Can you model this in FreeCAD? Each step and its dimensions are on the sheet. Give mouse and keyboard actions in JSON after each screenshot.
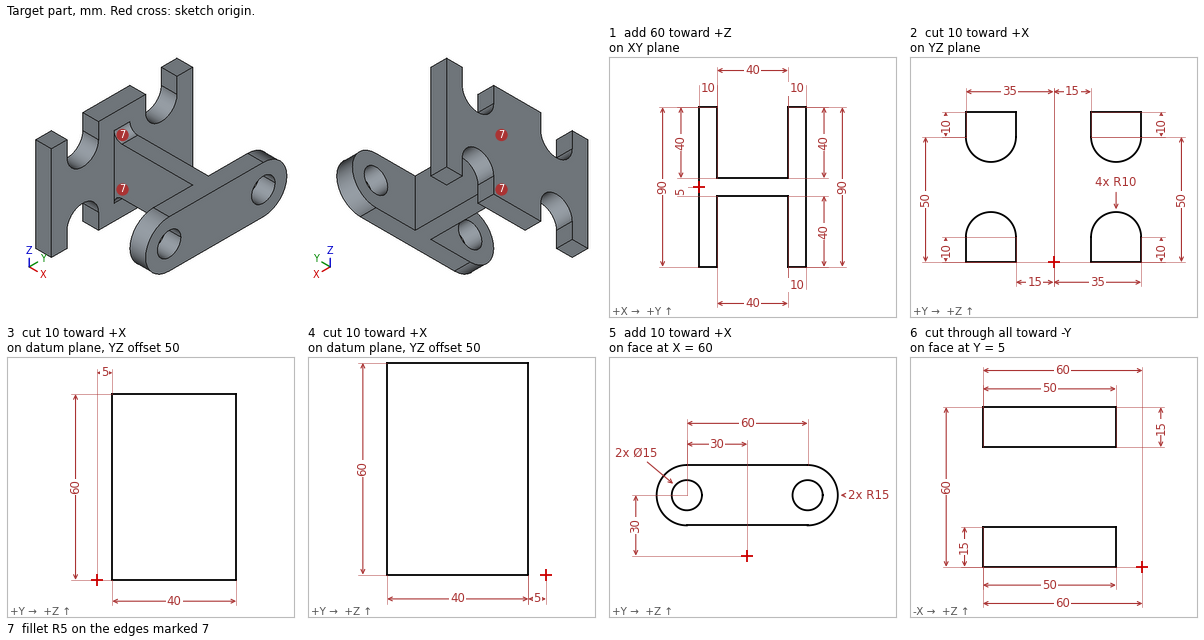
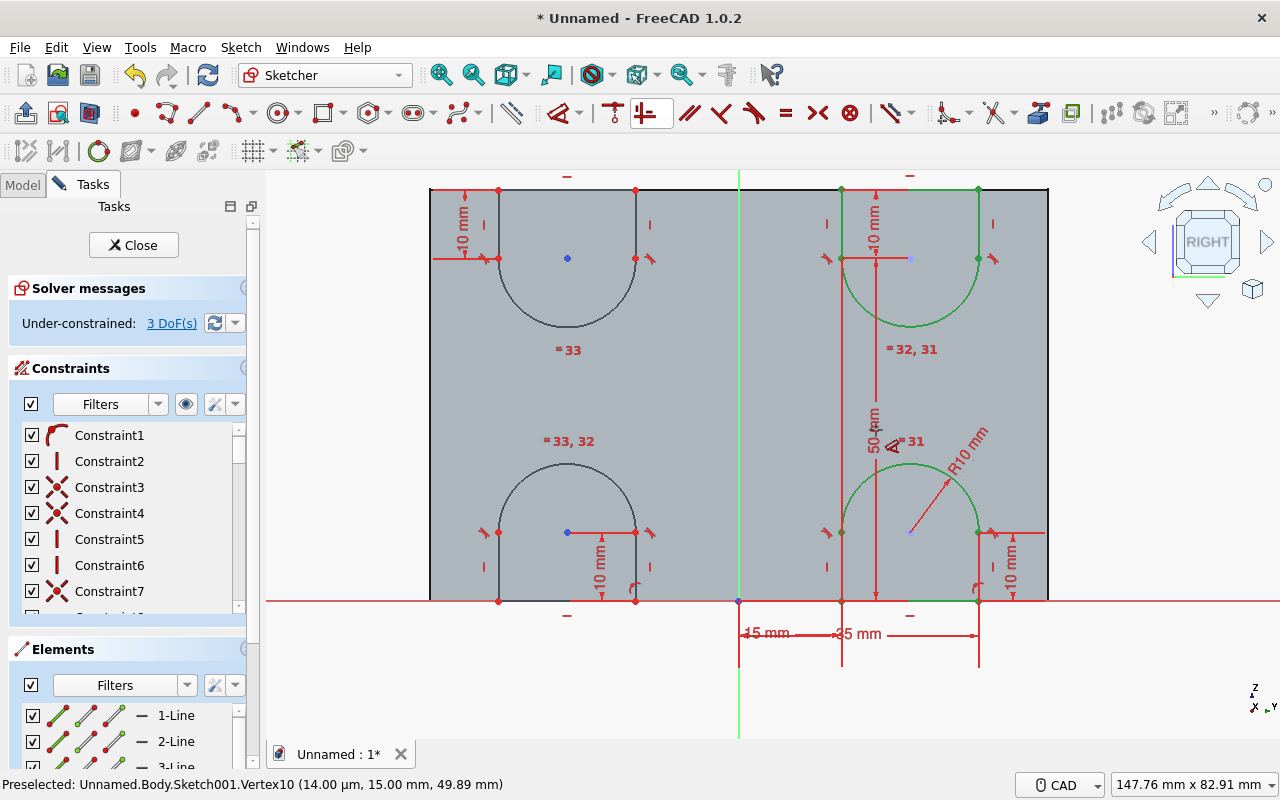
{"action": "left_click", "coordinate": [636, 533]}
{"action": "left_click", "coordinate": [687, 635]}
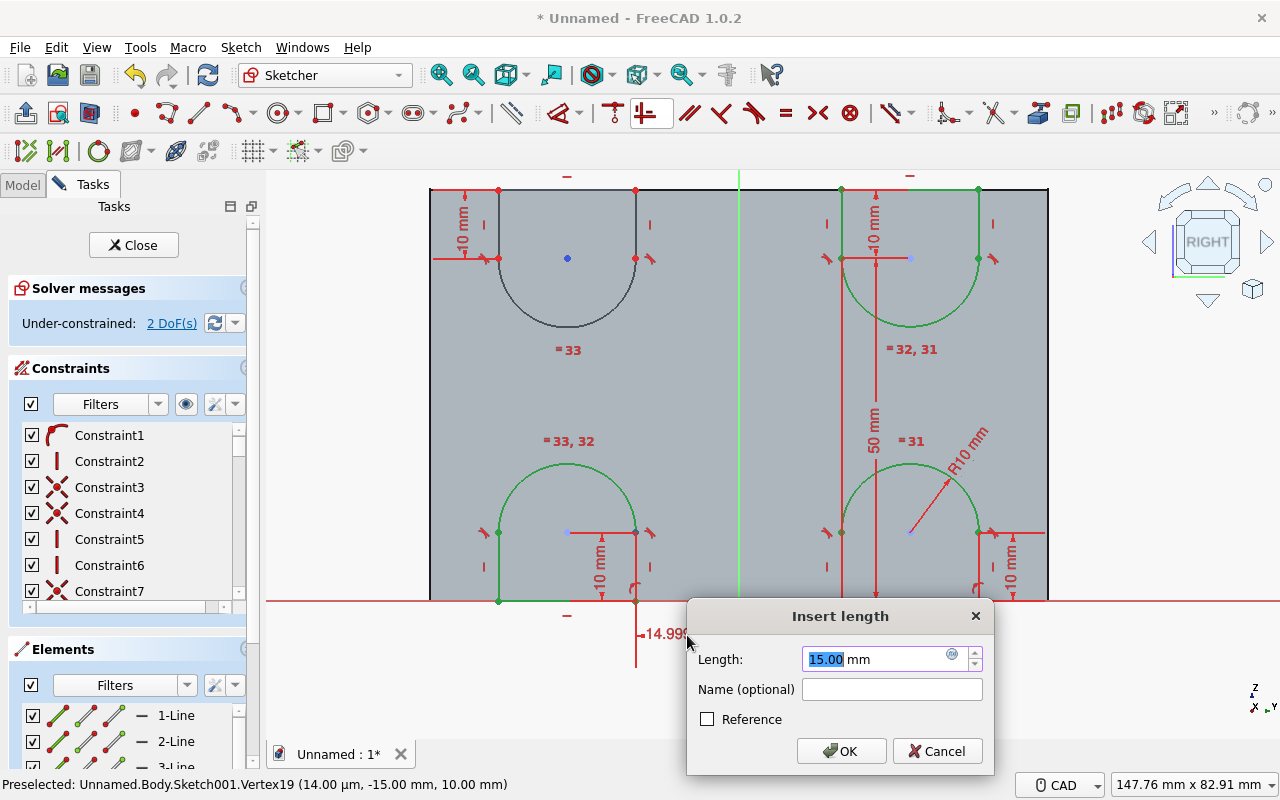
{"action": "type", "text": "15"}
{"action": "key", "text": "Return"}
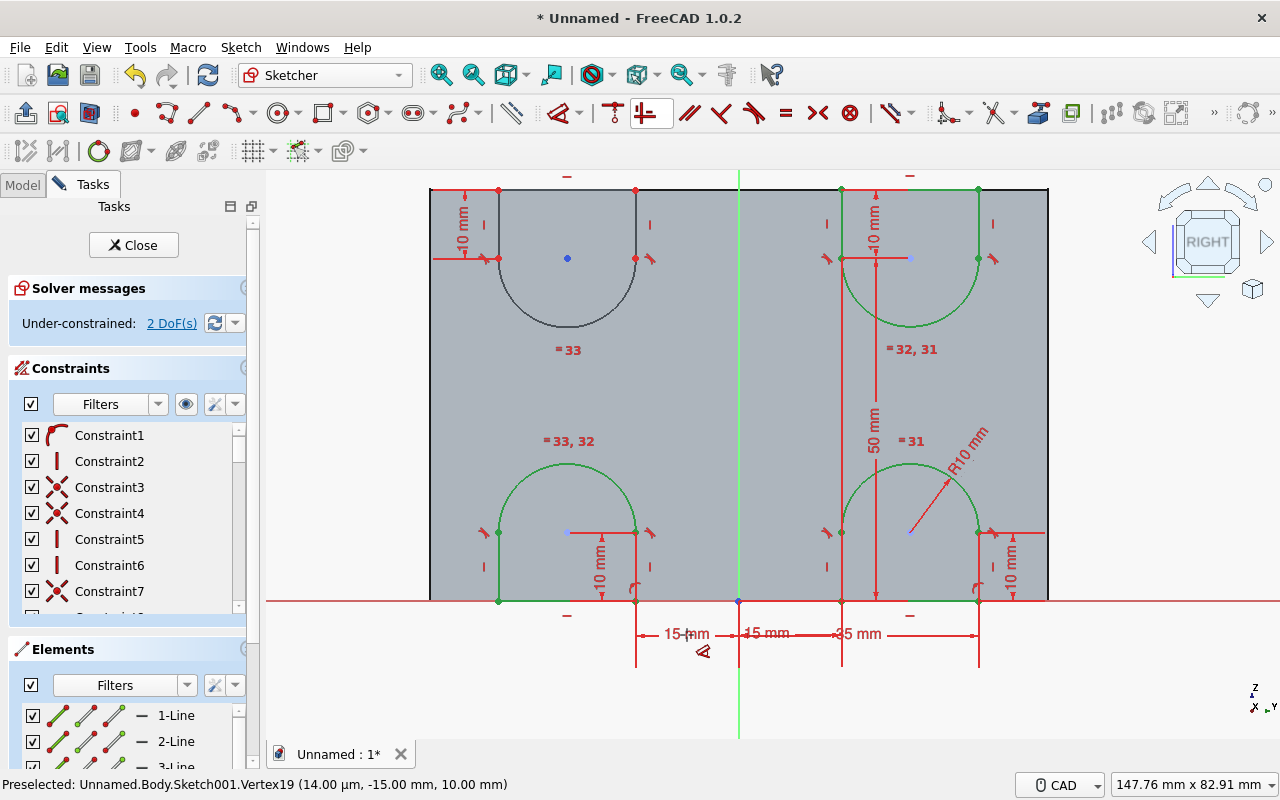
{"action": "left_click", "coordinate": [499, 259]}
{"action": "left_click", "coordinate": [563, 635]}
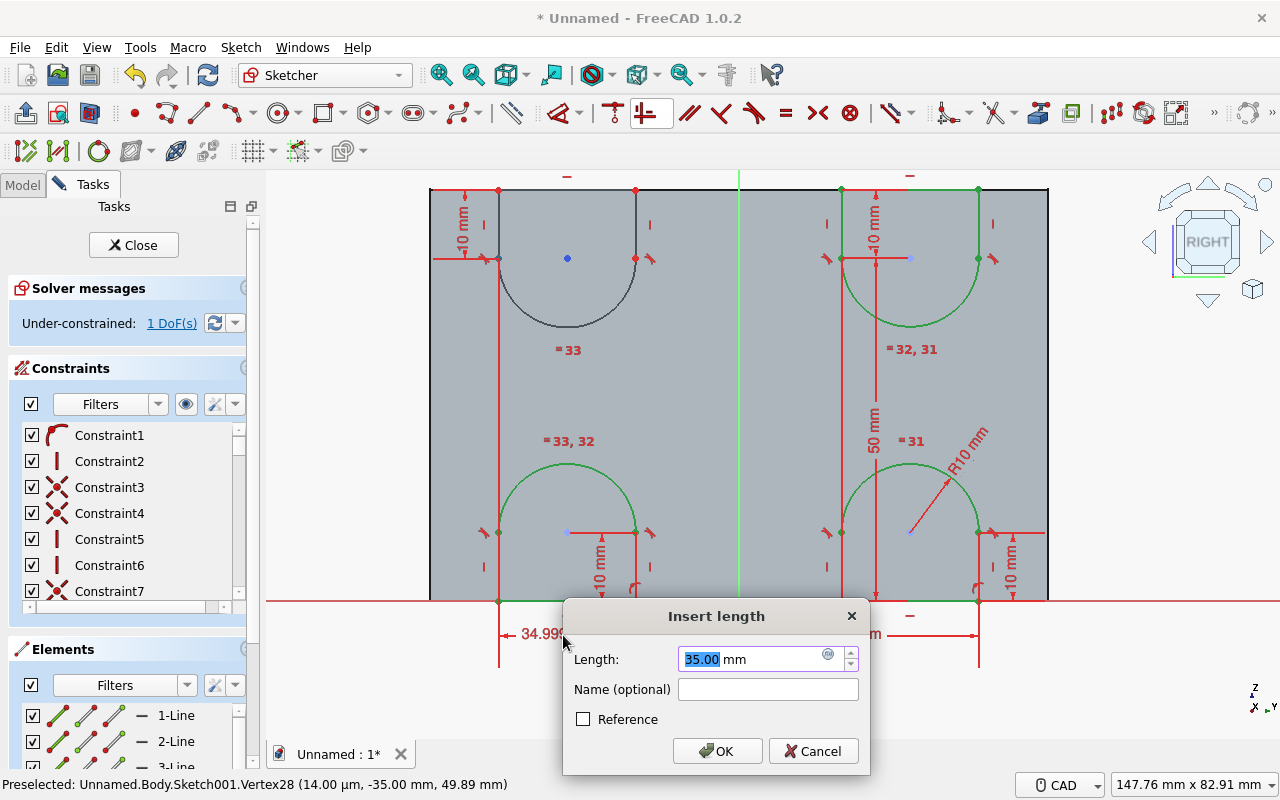
{"action": "type", "text": "35"}
{"action": "key", "text": "Return"}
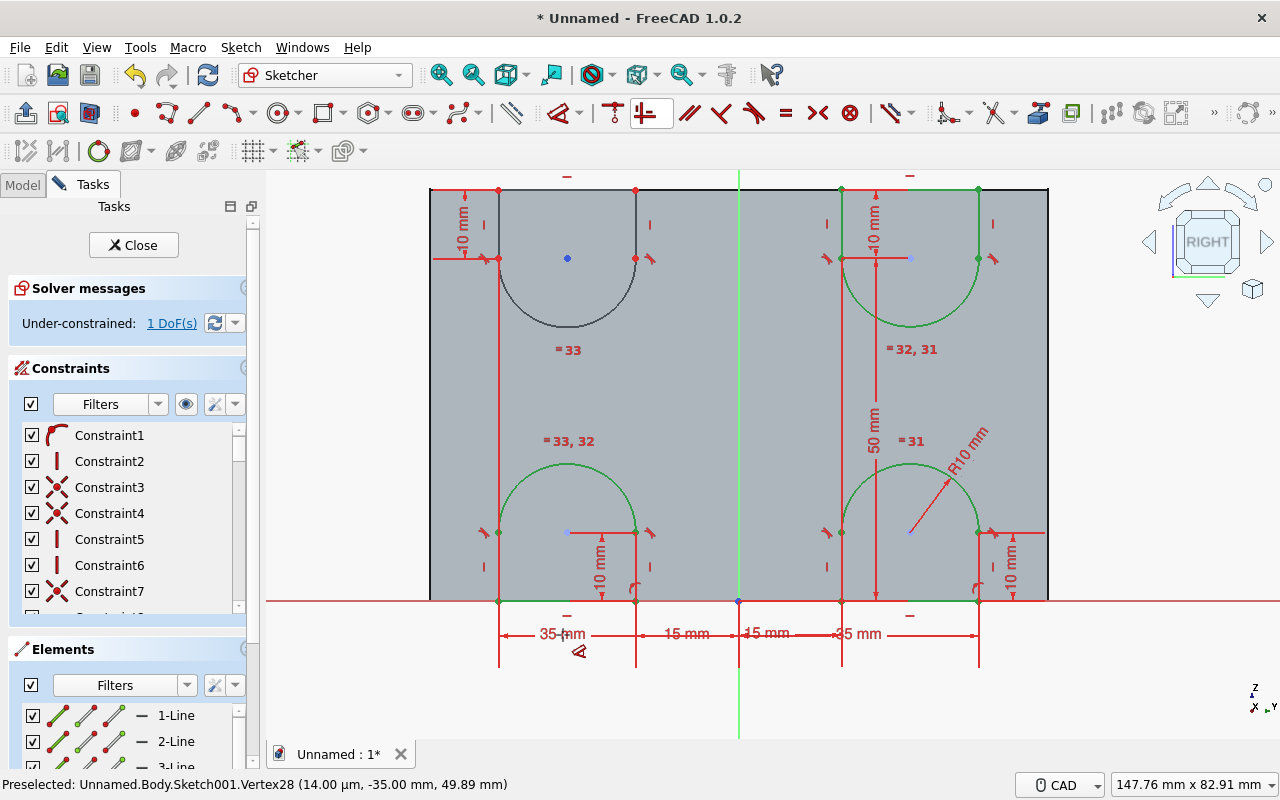
{"action": "left_click", "coordinate": [499, 259]}
{"action": "left_click", "coordinate": [465, 430]}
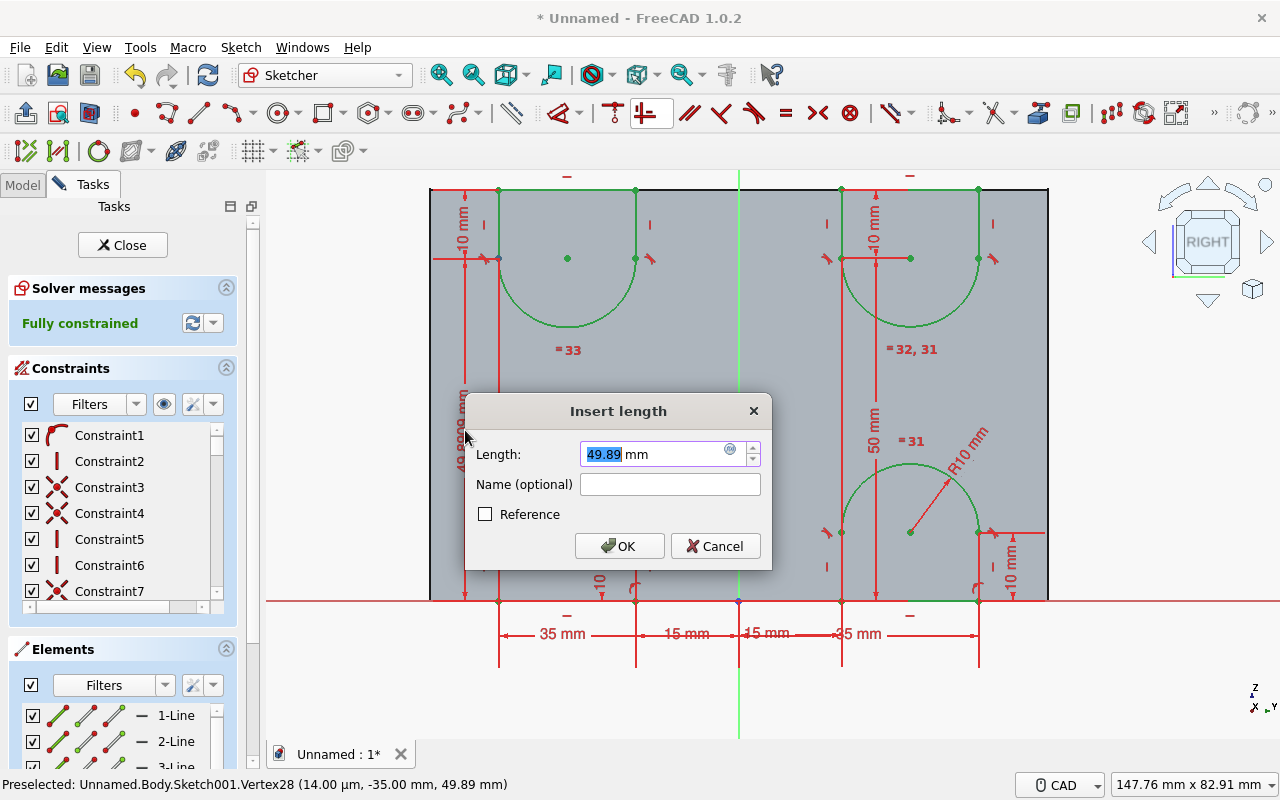
{"action": "type", "text": "50"}
{"action": "key", "text": "Return"}
{"action": "key", "text": "Escape"}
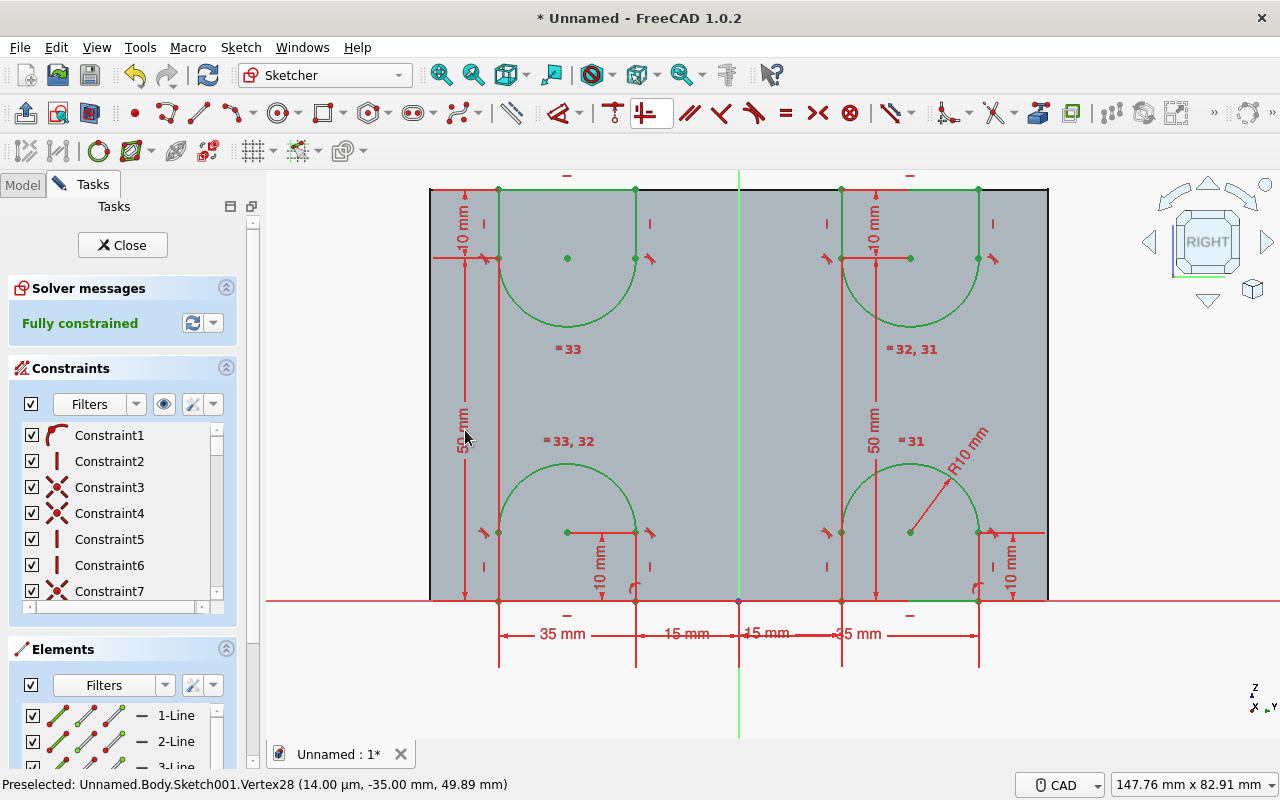
{"action": "left_click", "coordinate": [123, 245]}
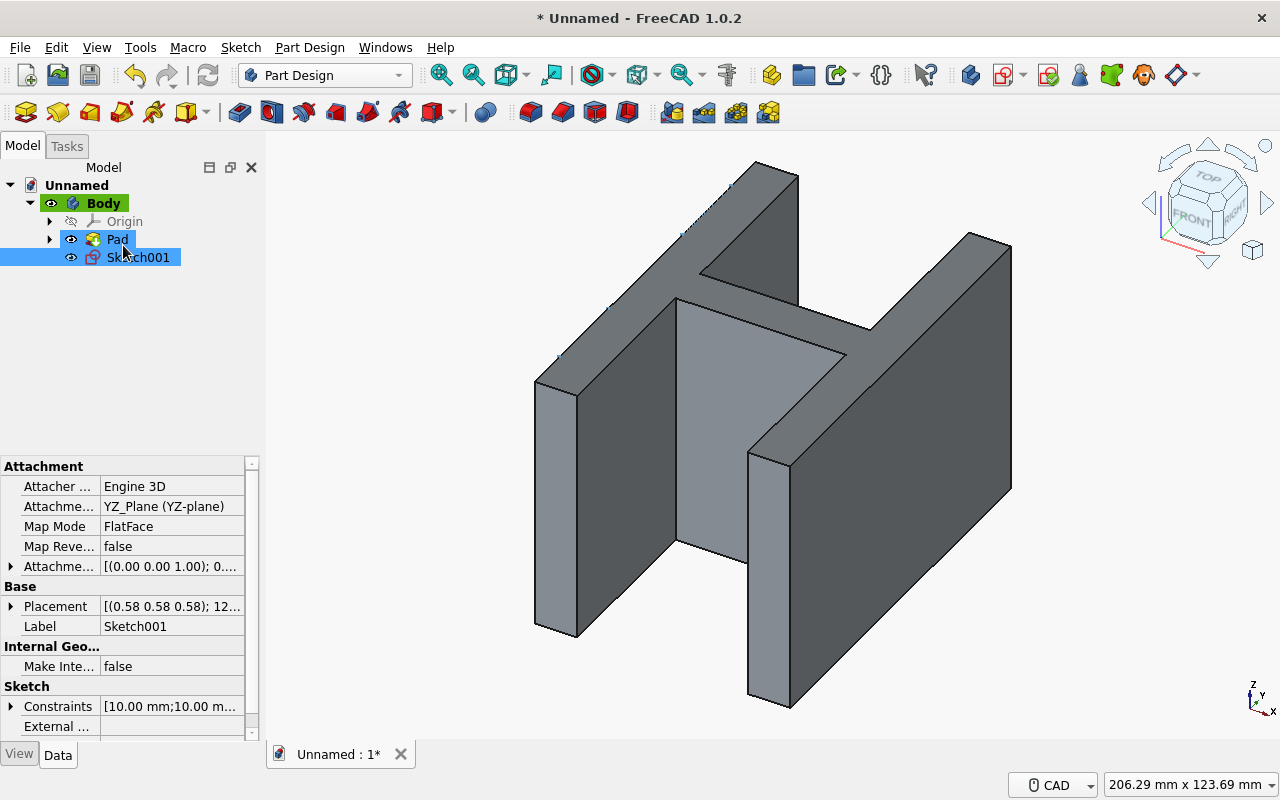
{"action": "left_click", "coordinate": [240, 112]}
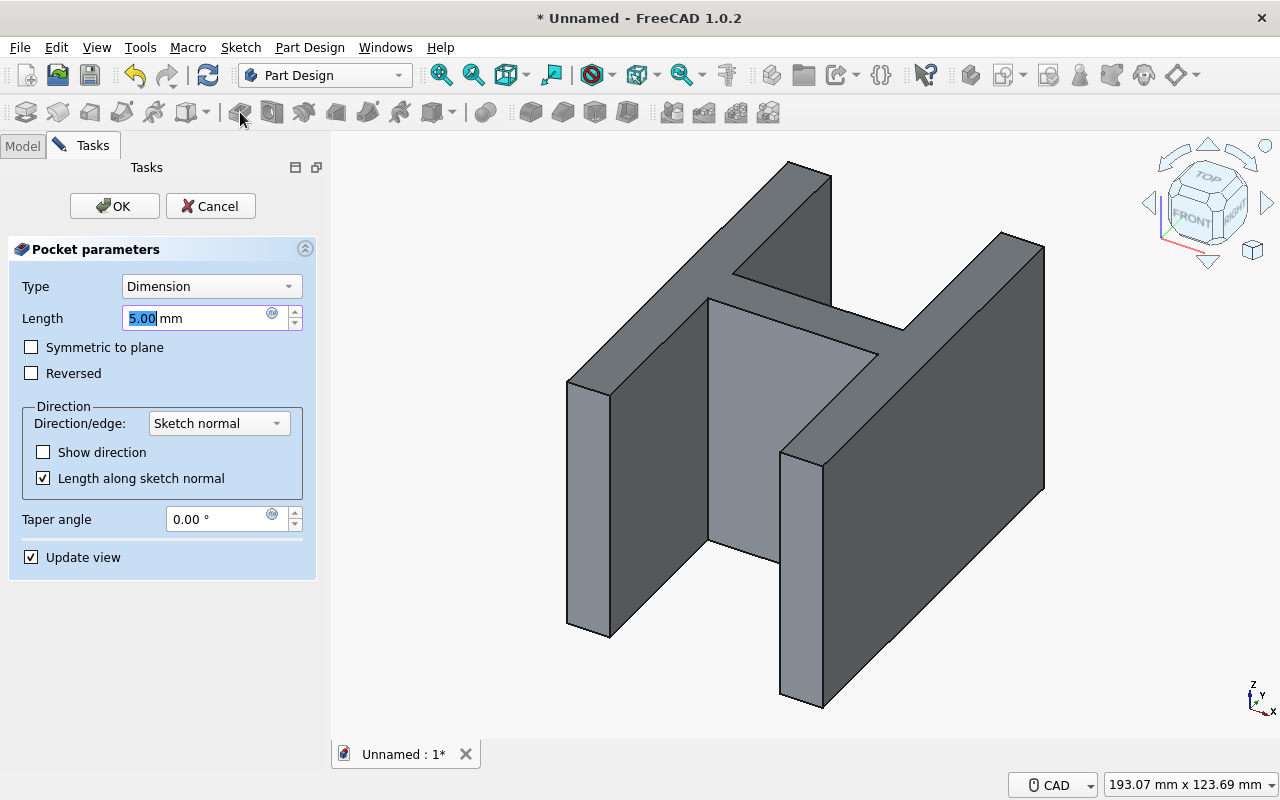
{"action": "type", "text": "10"}
{"action": "key", "text": "Tab"}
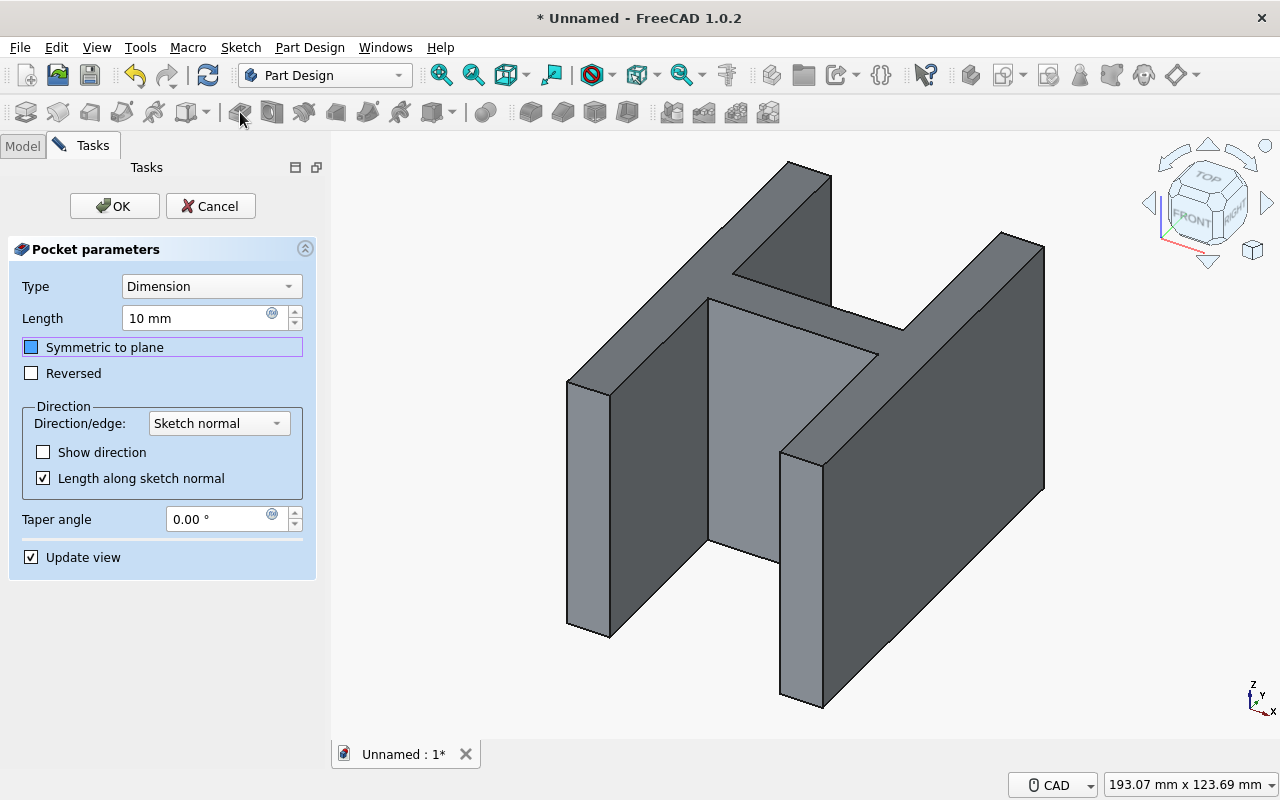
{"action": "left_click", "coordinate": [30, 373]}